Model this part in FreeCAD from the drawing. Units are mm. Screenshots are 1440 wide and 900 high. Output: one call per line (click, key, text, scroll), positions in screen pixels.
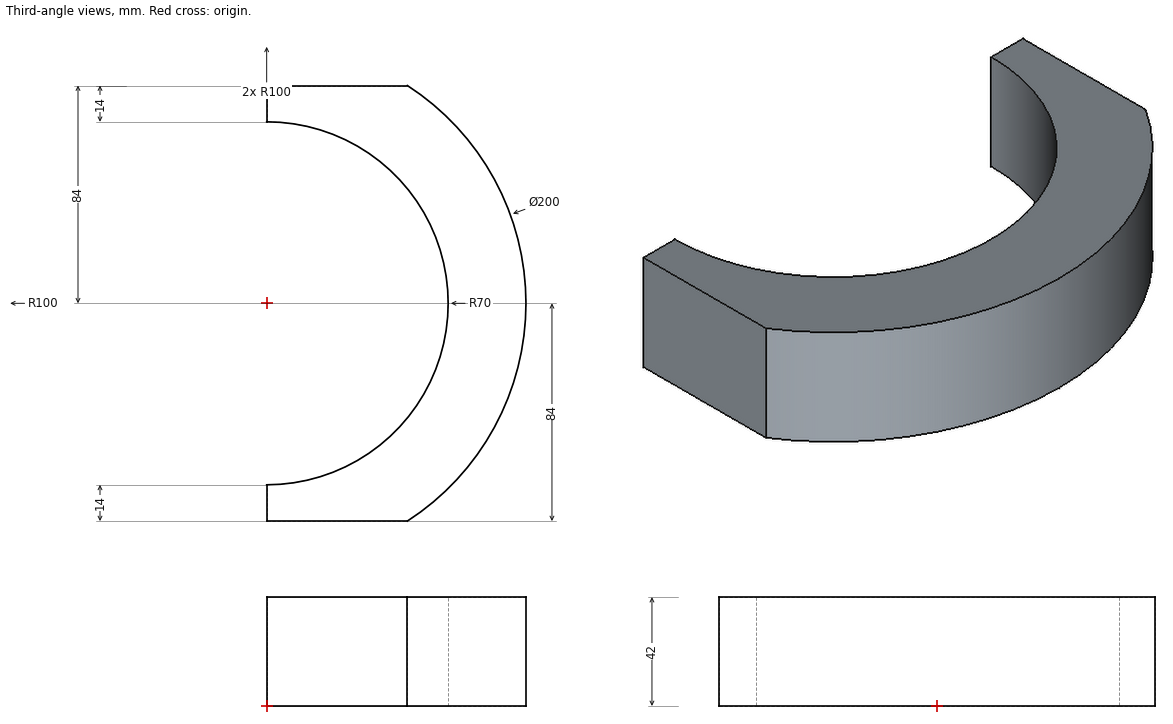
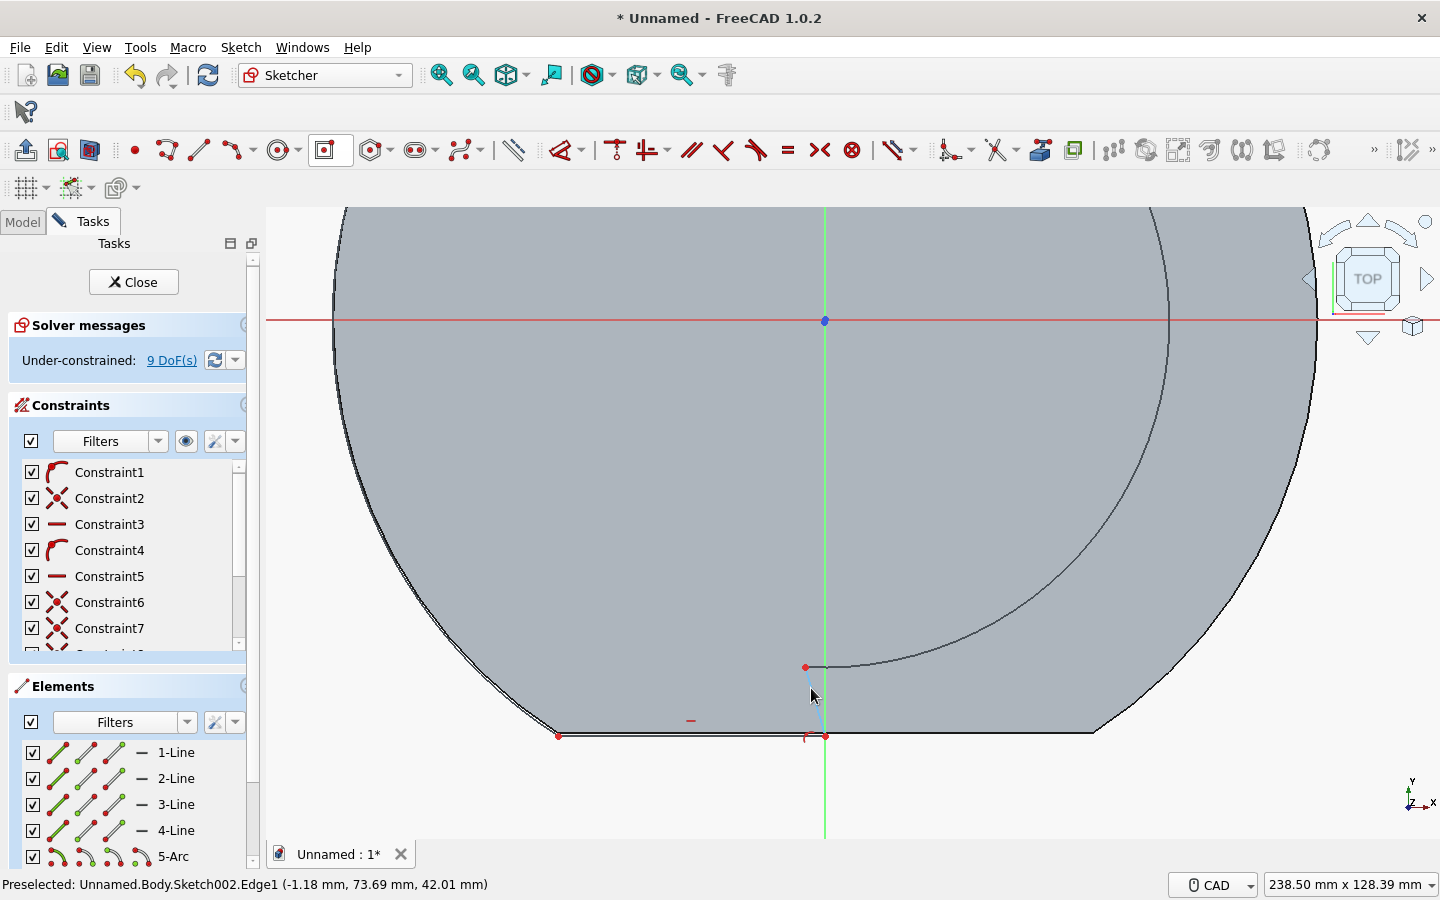
click(811, 688)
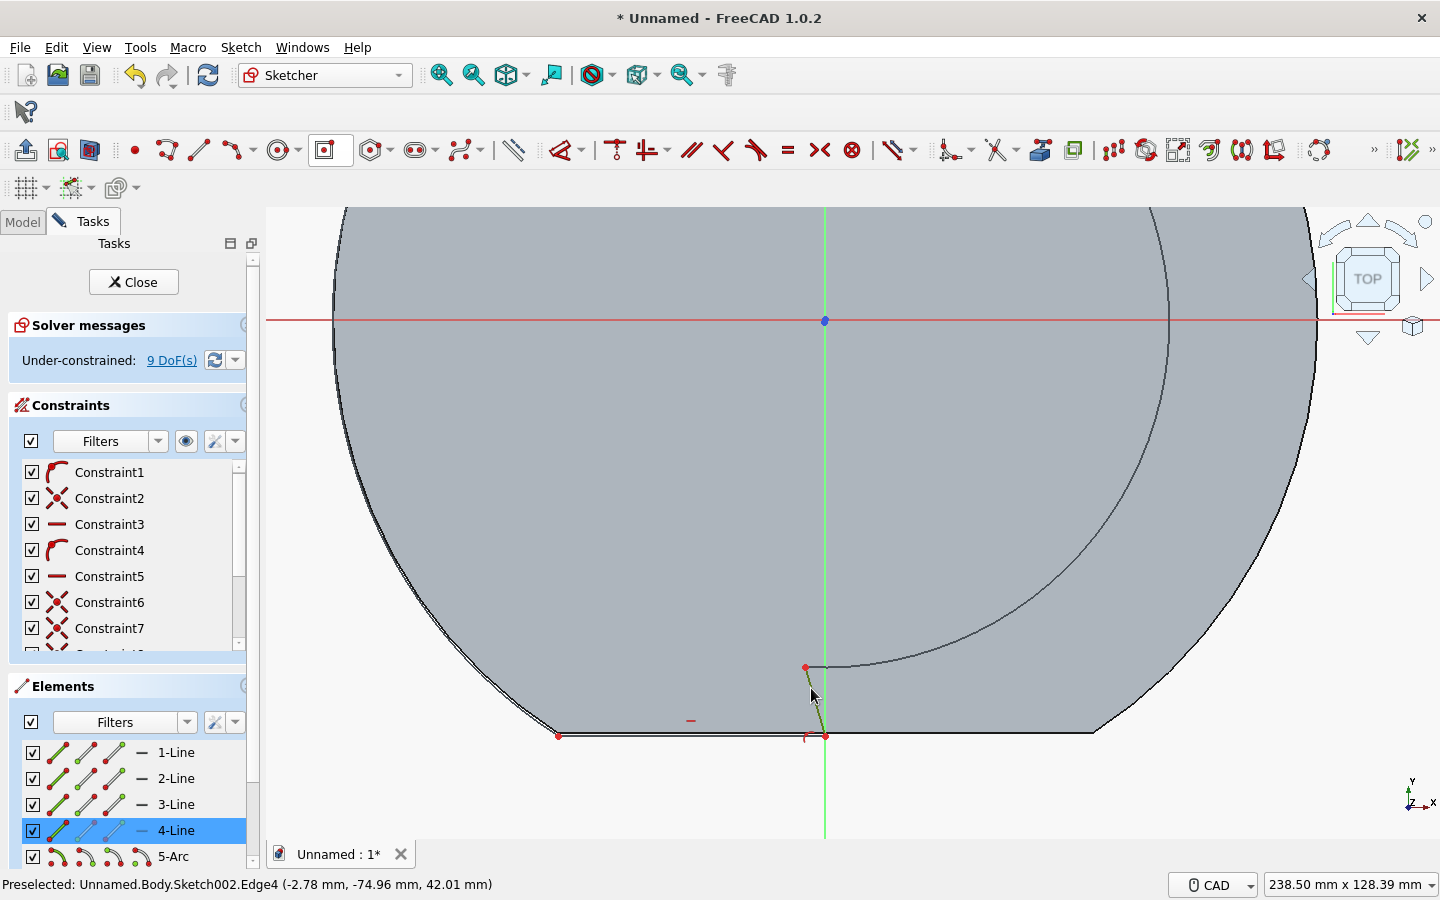
key(v)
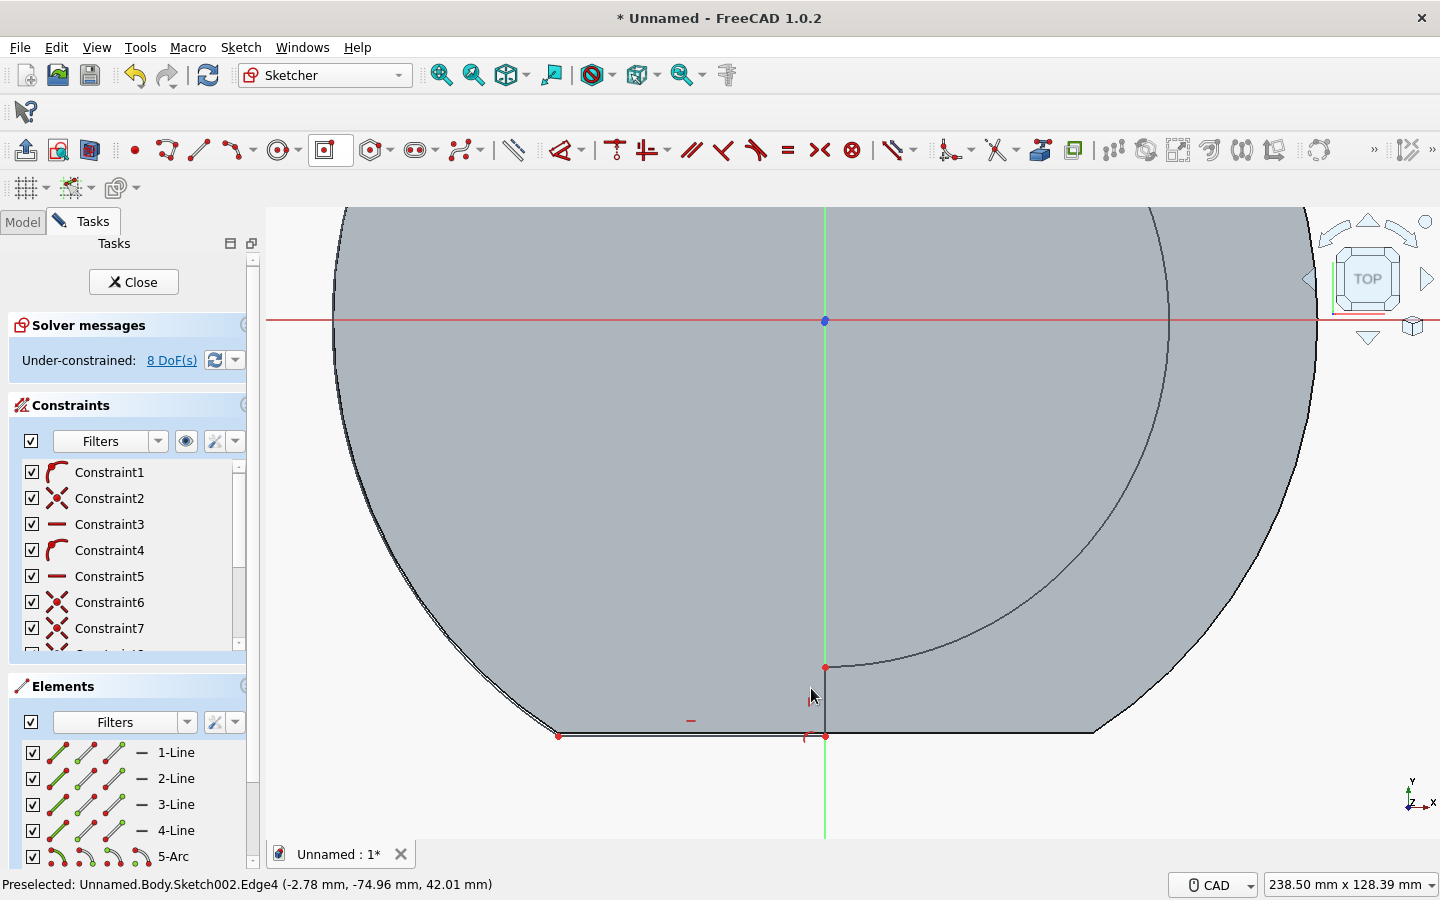
click(371, 514)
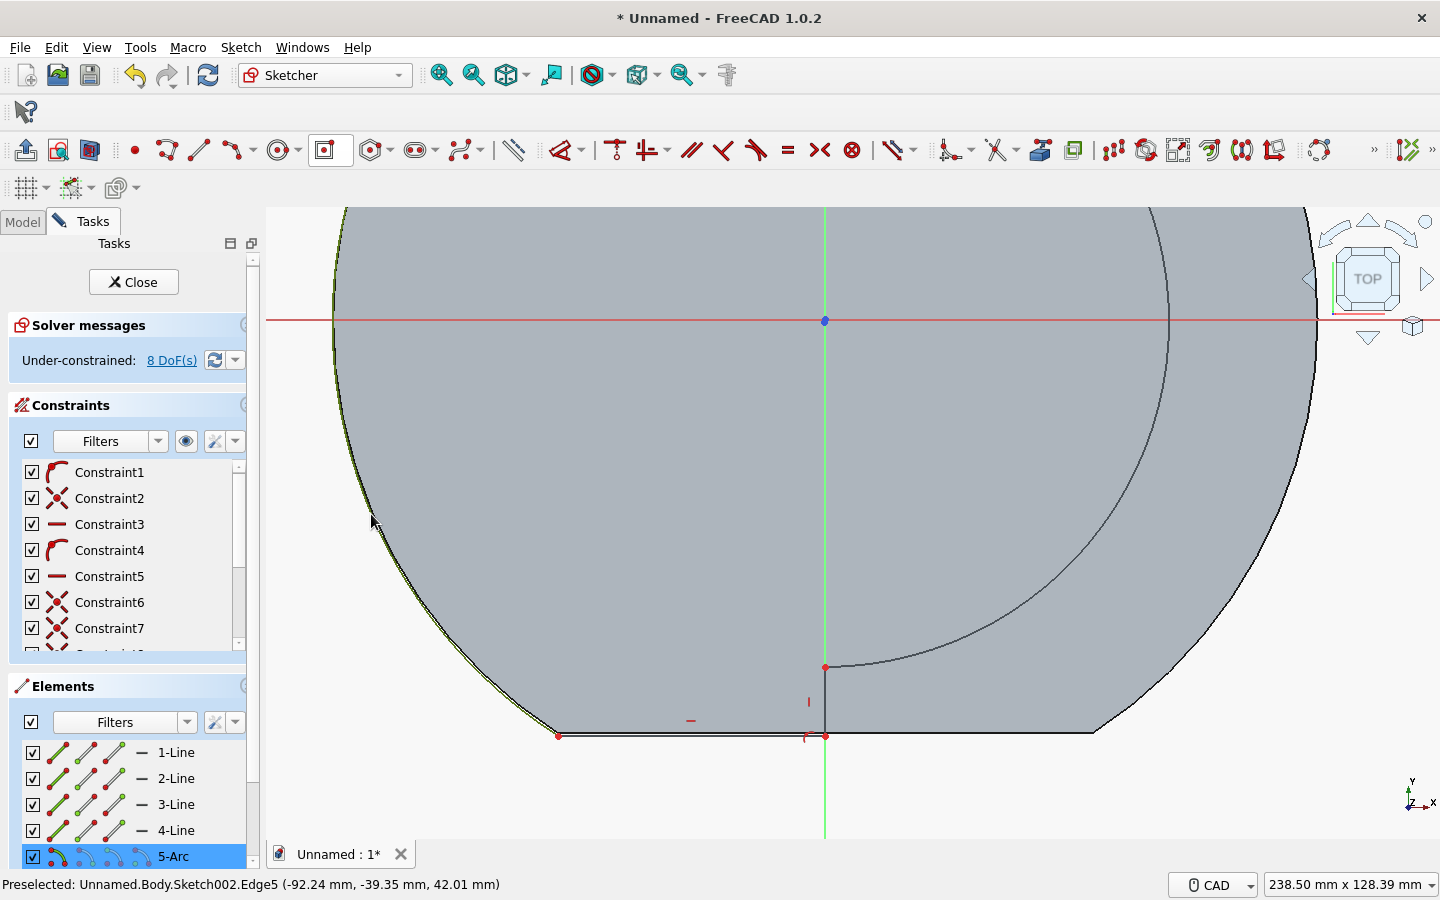
click(1103, 524)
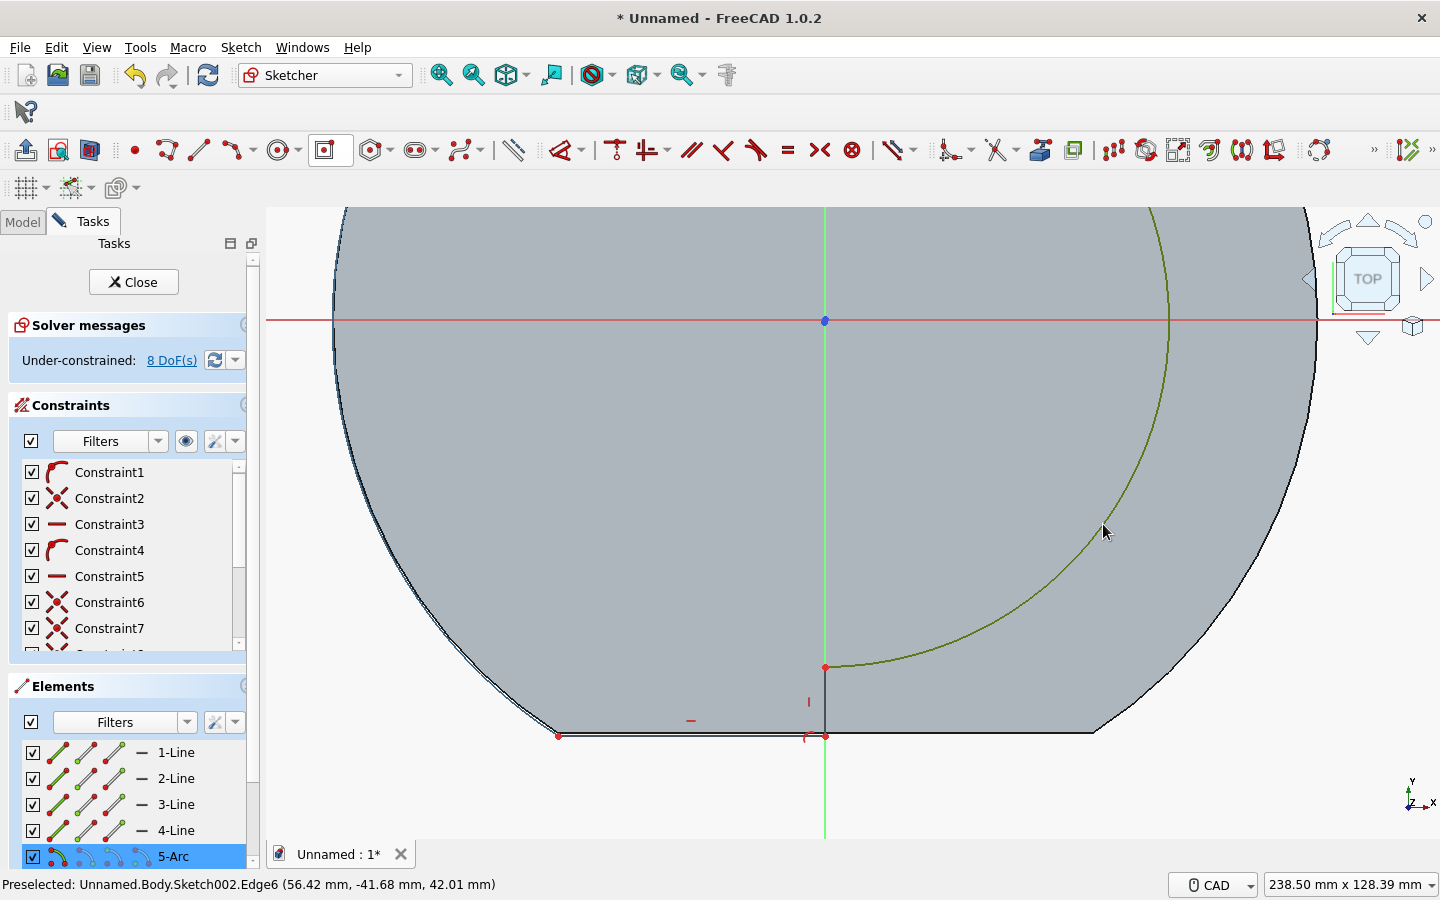
click(616, 150)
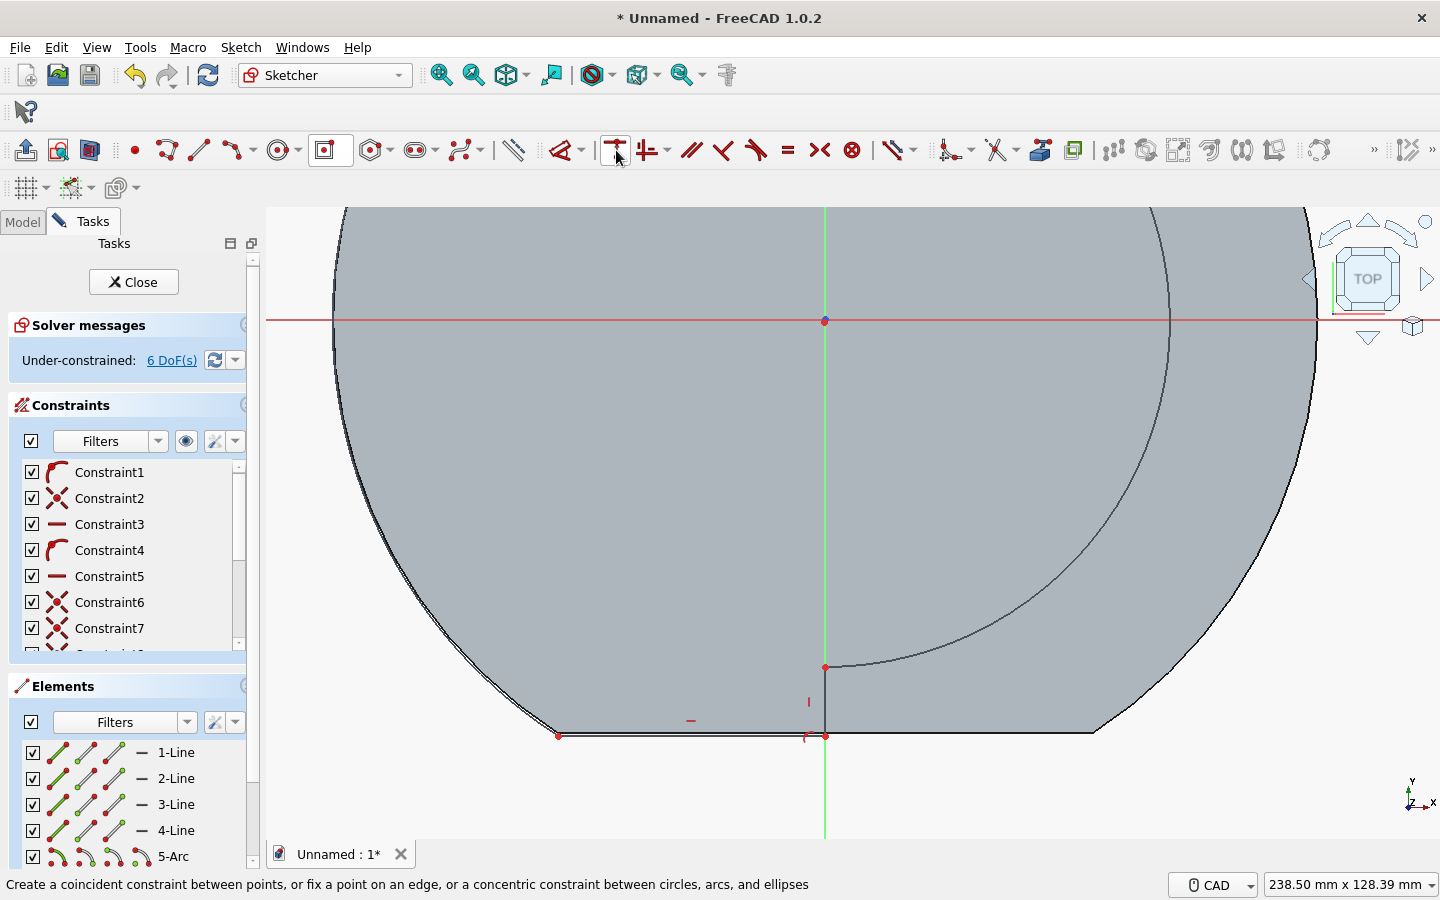
drag(815, 310, 835, 332)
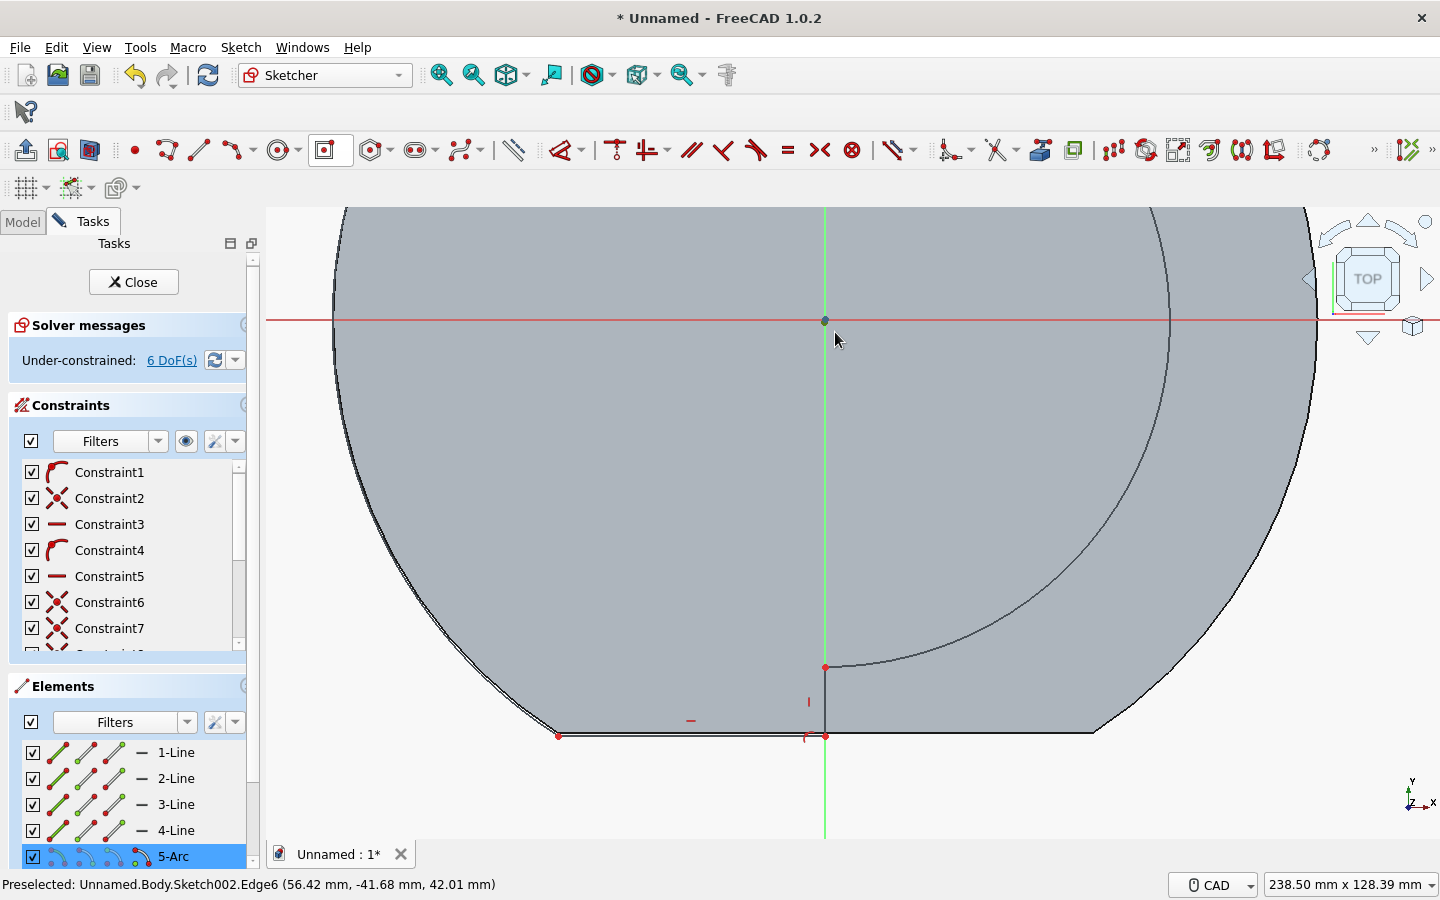
click(616, 150)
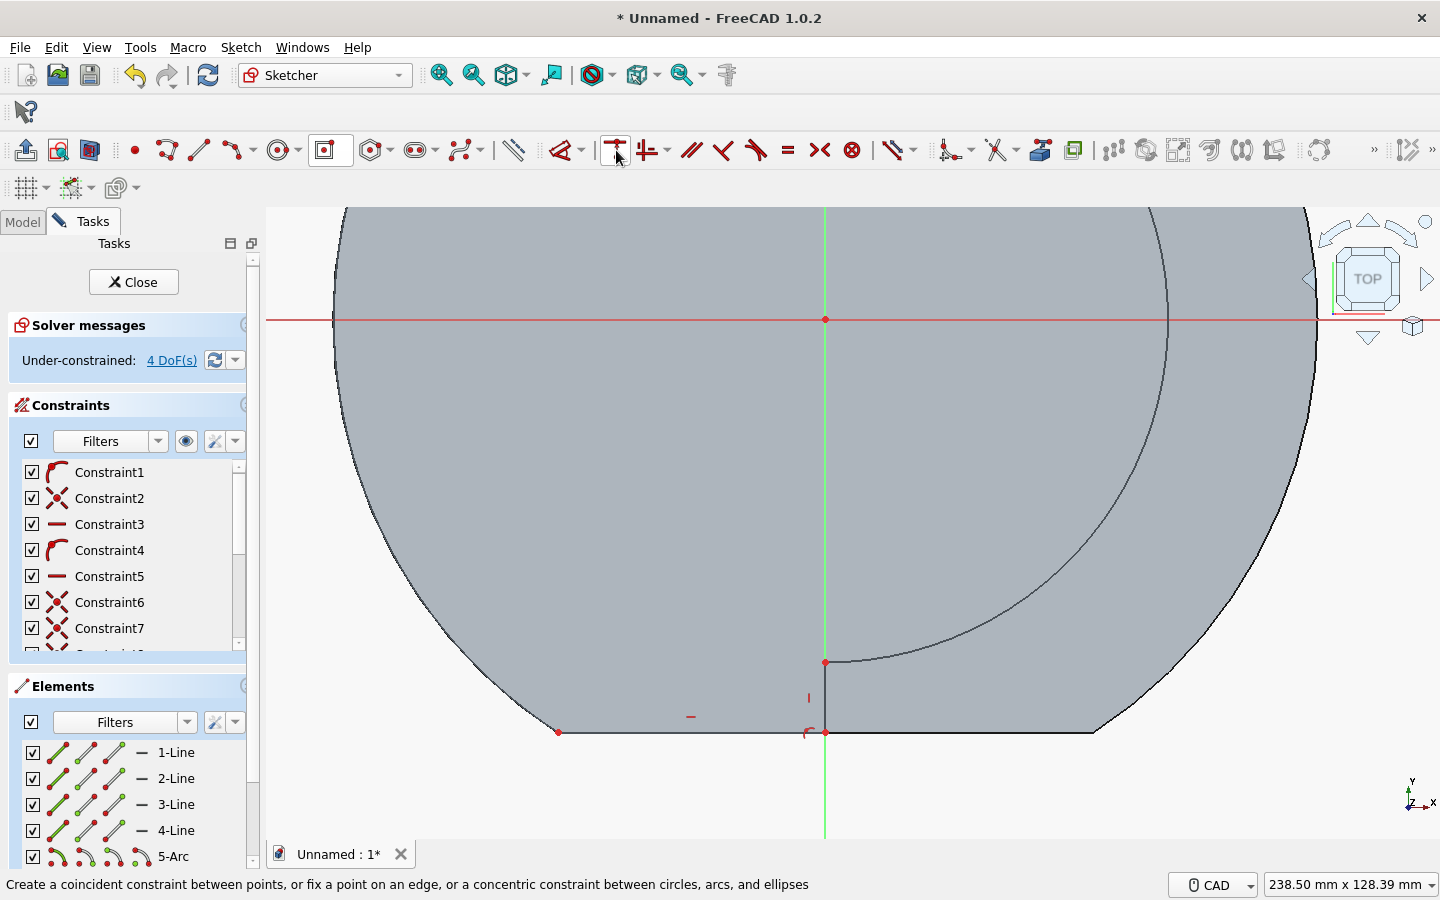
click(560, 150)